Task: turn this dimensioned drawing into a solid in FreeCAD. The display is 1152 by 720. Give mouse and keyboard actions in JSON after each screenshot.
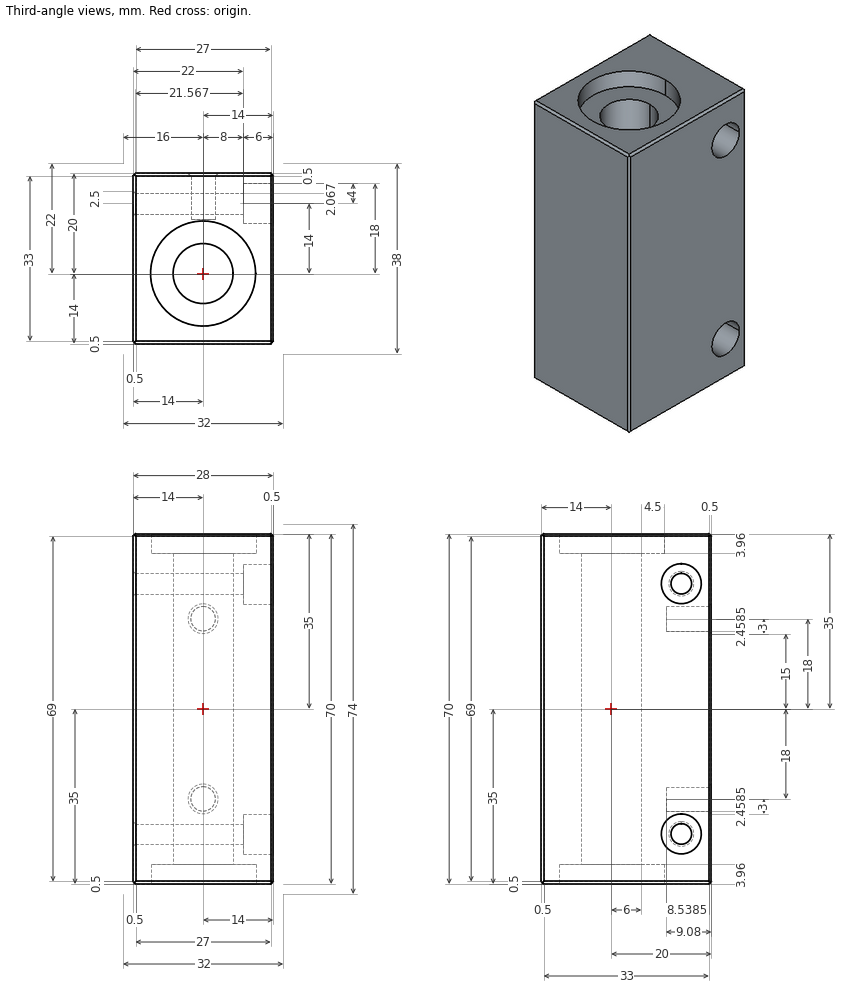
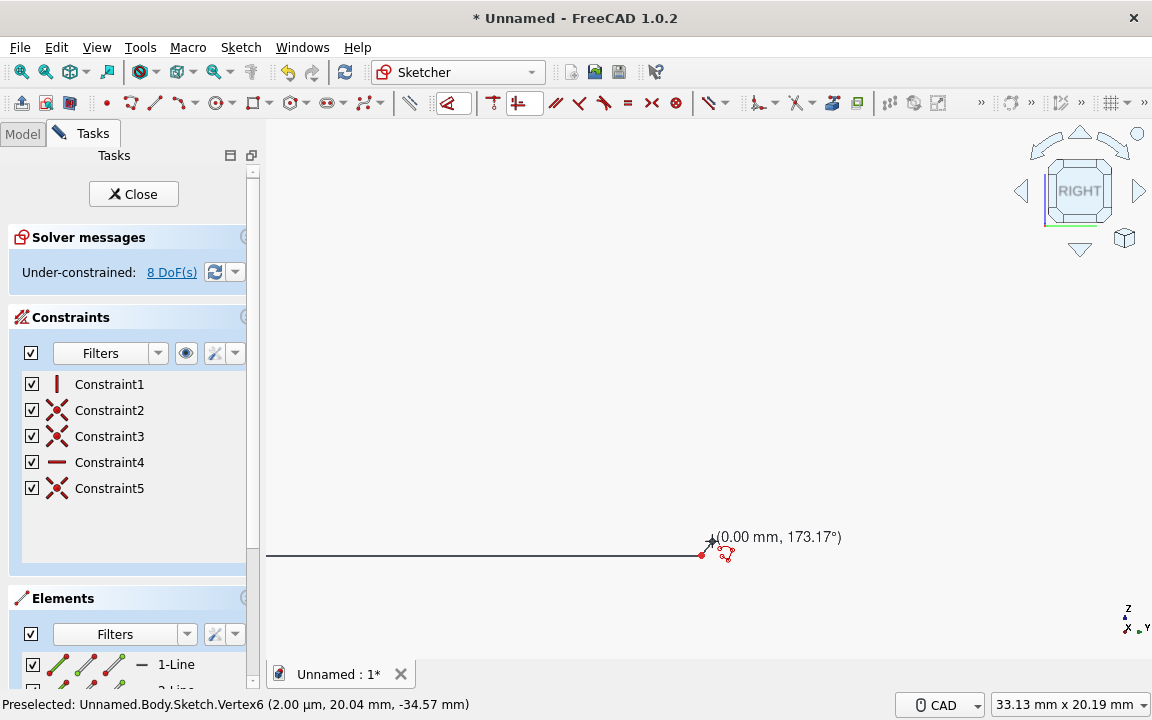
{"action": "scroll", "coordinate": [716, 542], "scroll_direction": "down", "scroll_amount": 9}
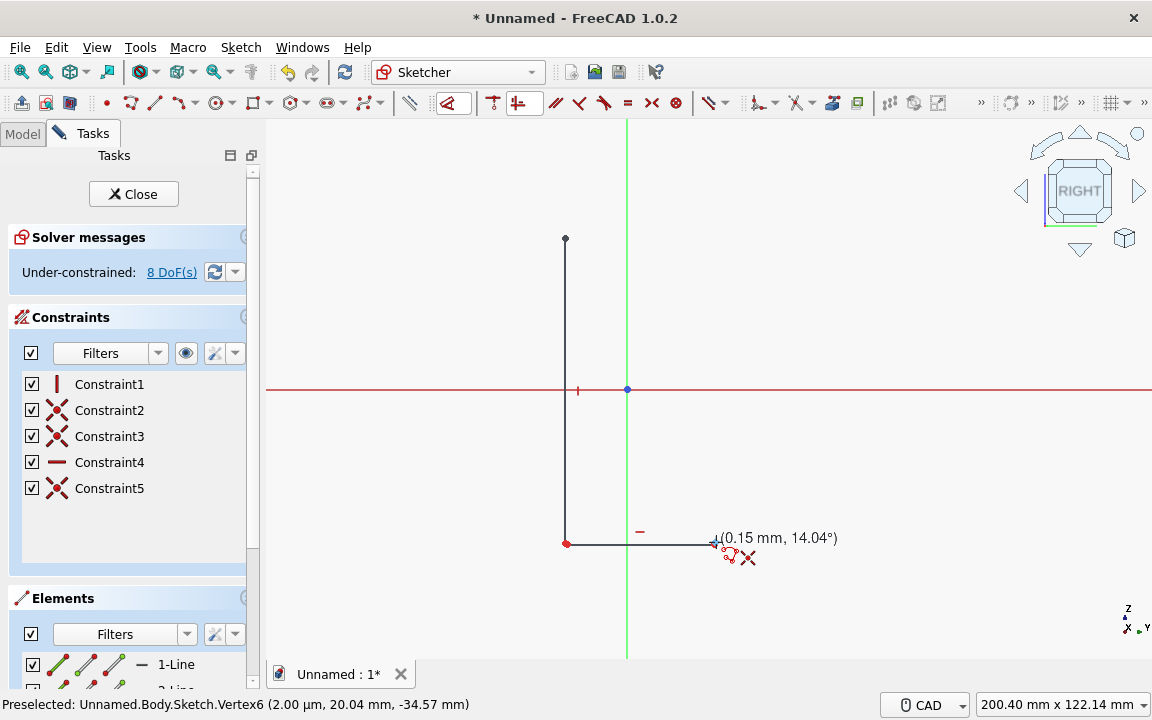
{"action": "left_click", "coordinate": [716, 237]}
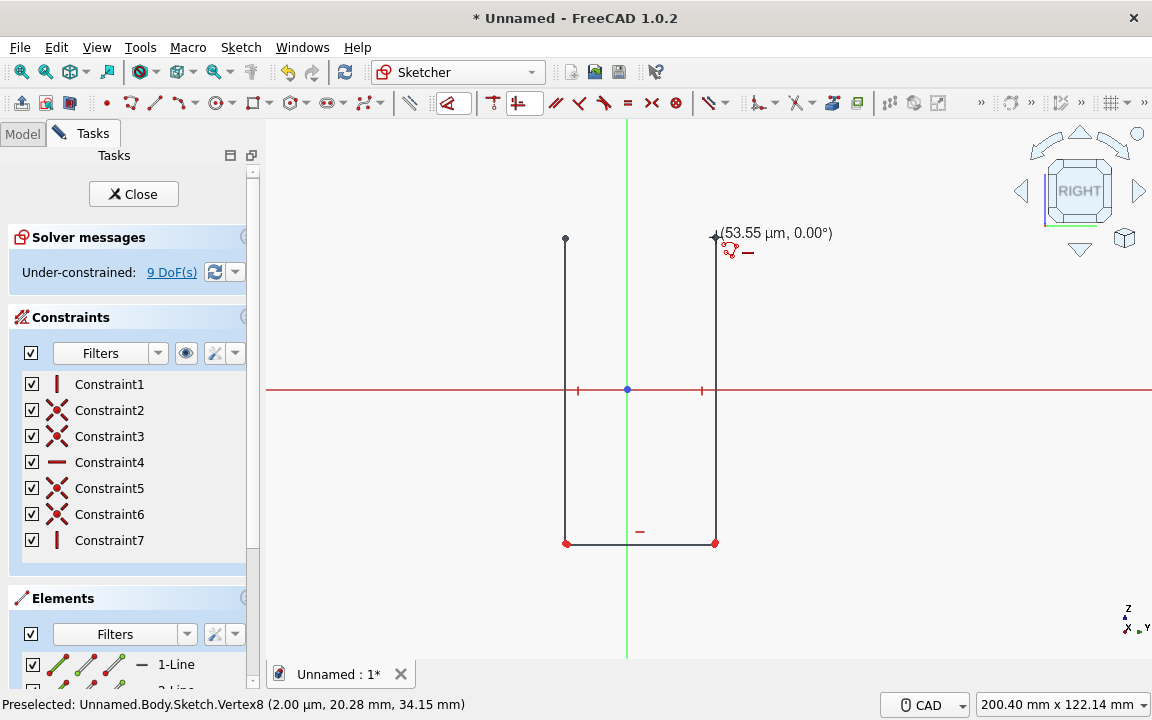
{"action": "scroll", "coordinate": [714, 235], "scroll_direction": "up", "scroll_amount": 9}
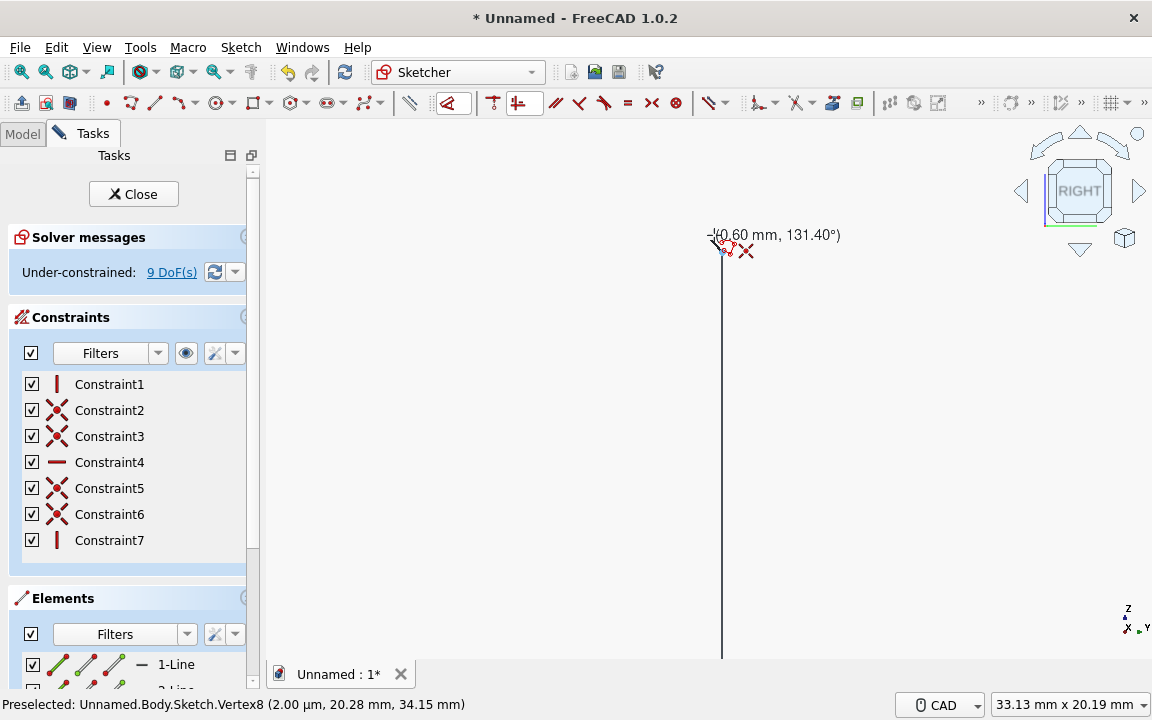
{"action": "left_click", "coordinate": [709, 235]}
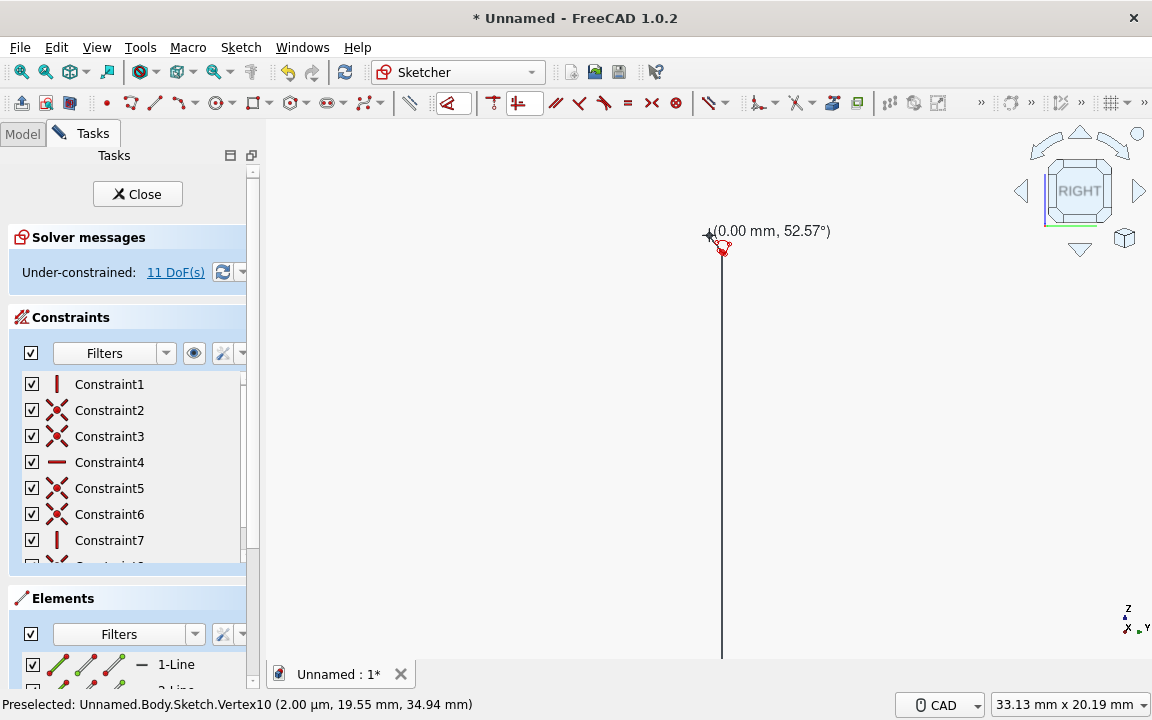
{"action": "scroll", "coordinate": [714, 234], "scroll_direction": "down", "scroll_amount": 9}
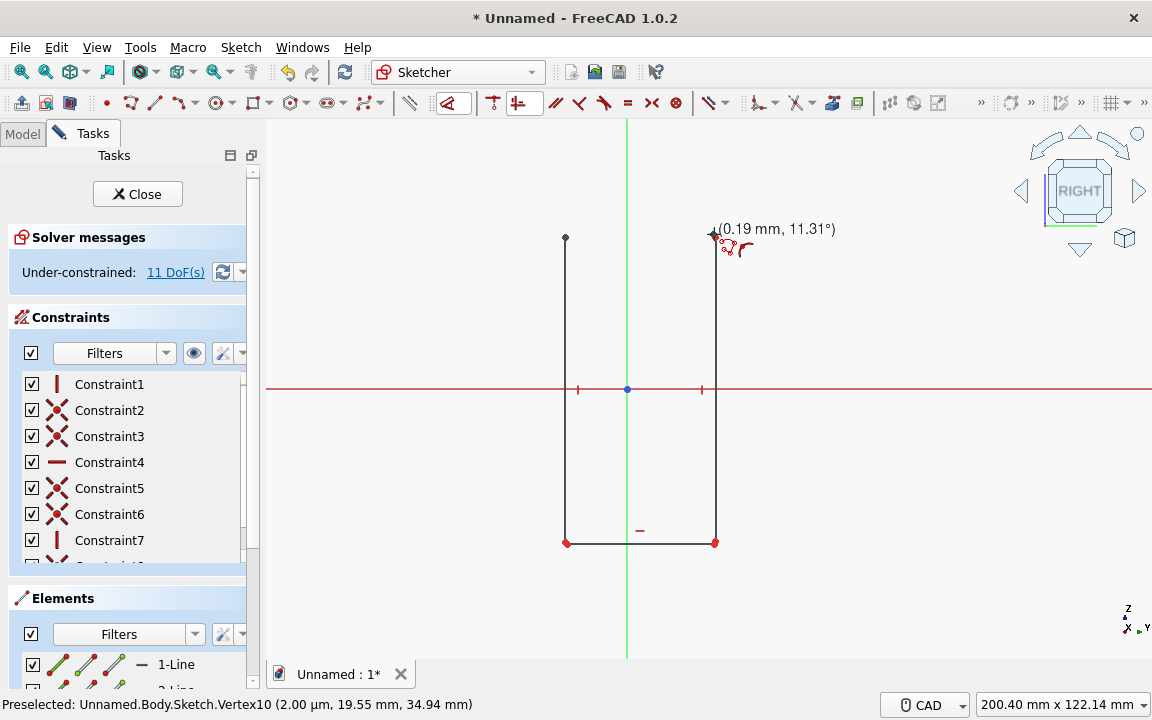
{"action": "scroll", "coordinate": [568, 234], "scroll_direction": "up", "scroll_amount": 9}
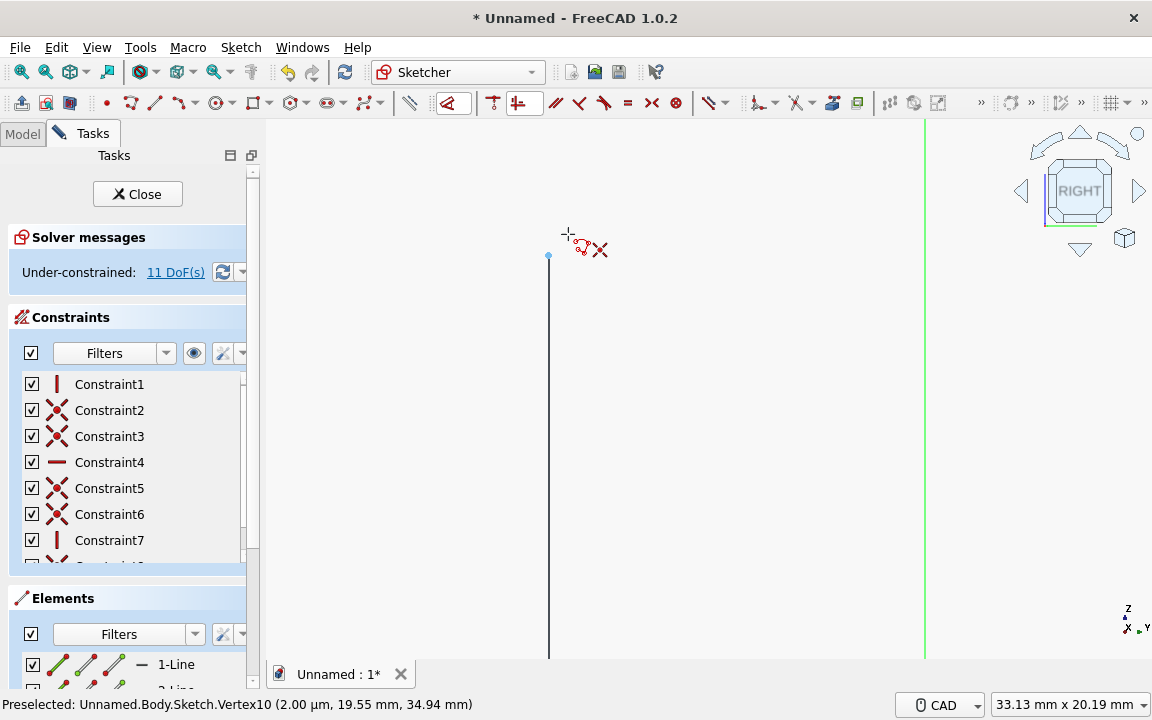
{"action": "left_click", "coordinate": [564, 235]}
{"action": "left_click", "coordinate": [549, 255]}
{"action": "key", "text": "Escape"}
{"action": "key", "text": "Escape"}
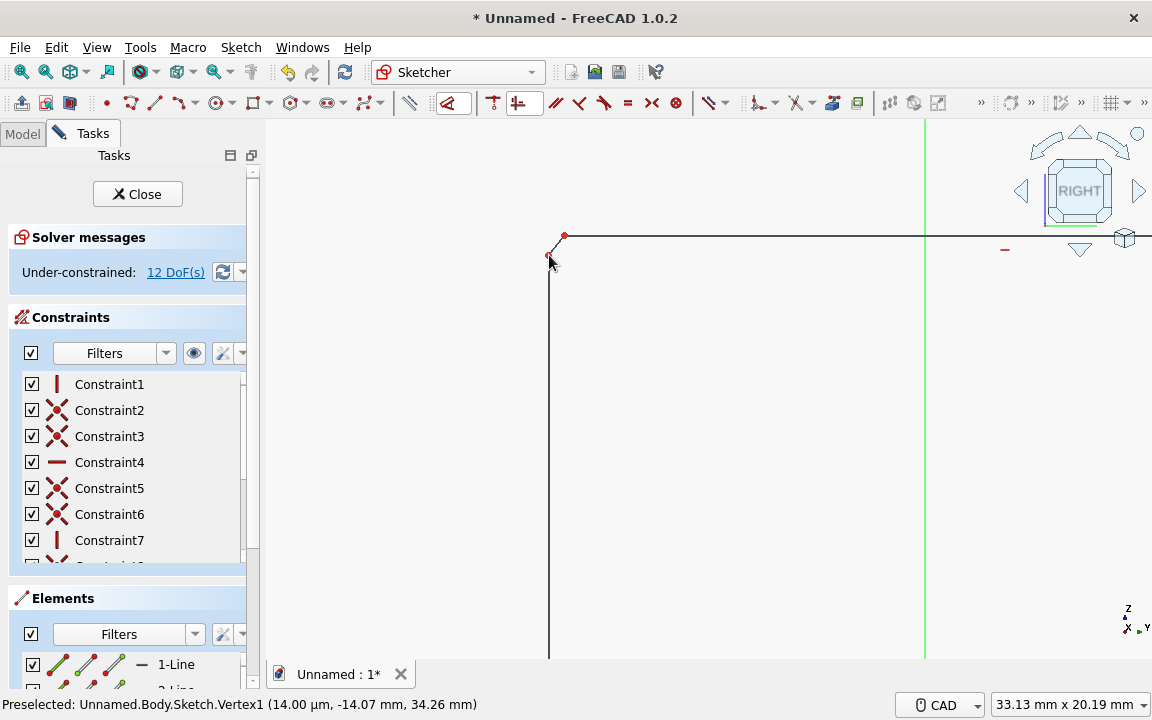
{"action": "left_click", "coordinate": [448, 104]}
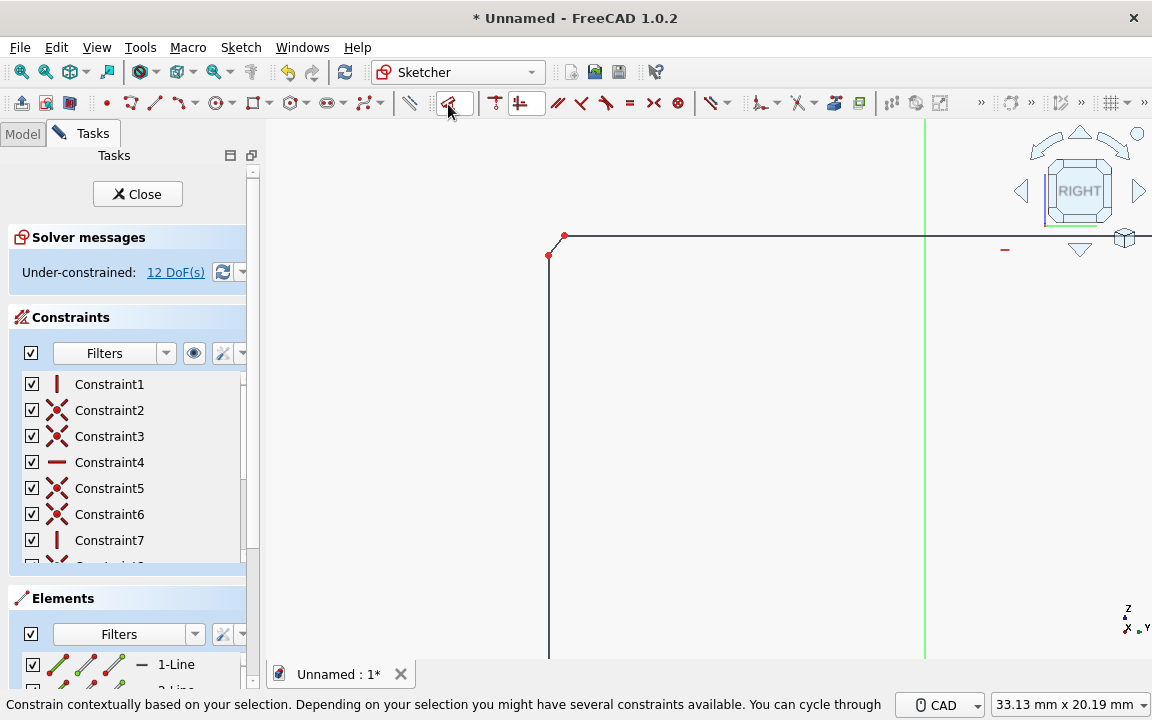
{"action": "scroll", "coordinate": [568, 234], "scroll_direction": "down", "scroll_amount": 9}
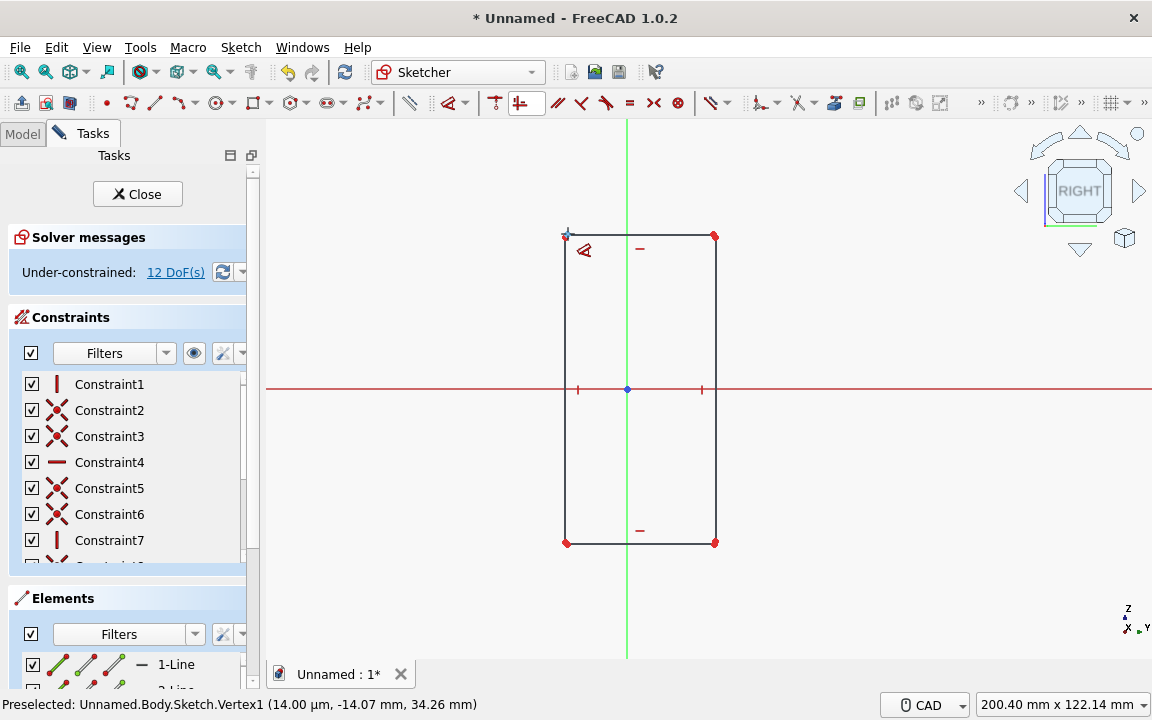
{"action": "left_click", "coordinate": [565, 299]}
{"action": "left_click", "coordinate": [531, 320]}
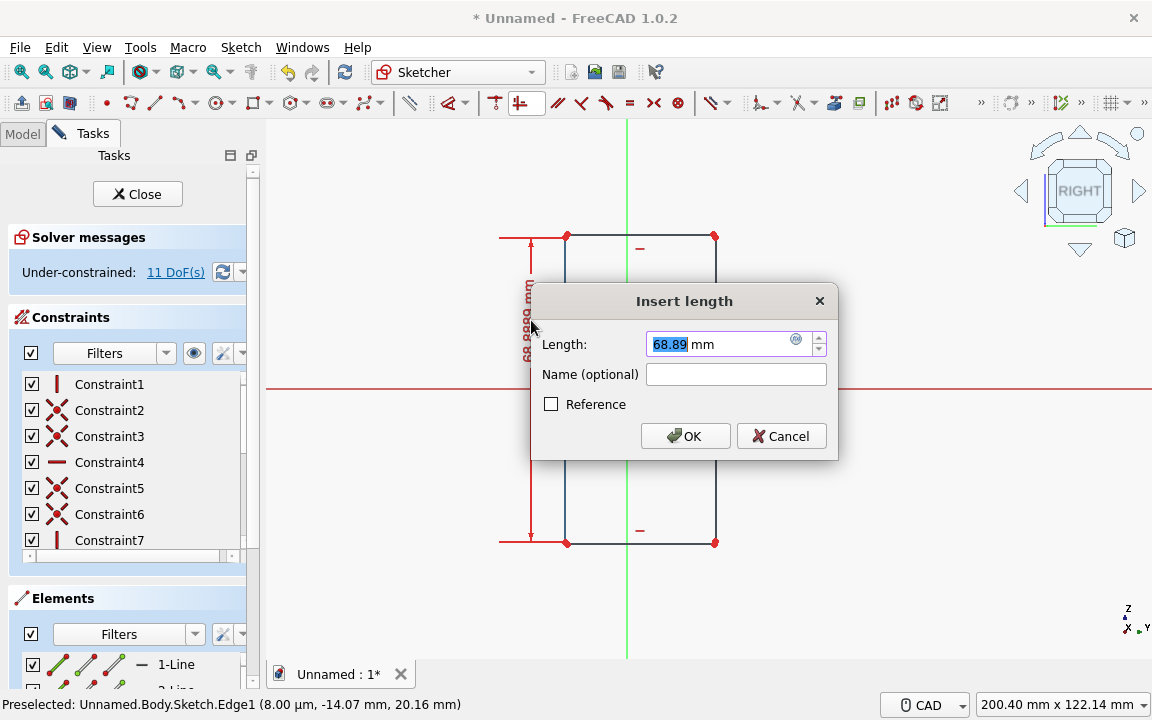
{"action": "type", "text": "69"}
{"action": "key", "text": "Return"}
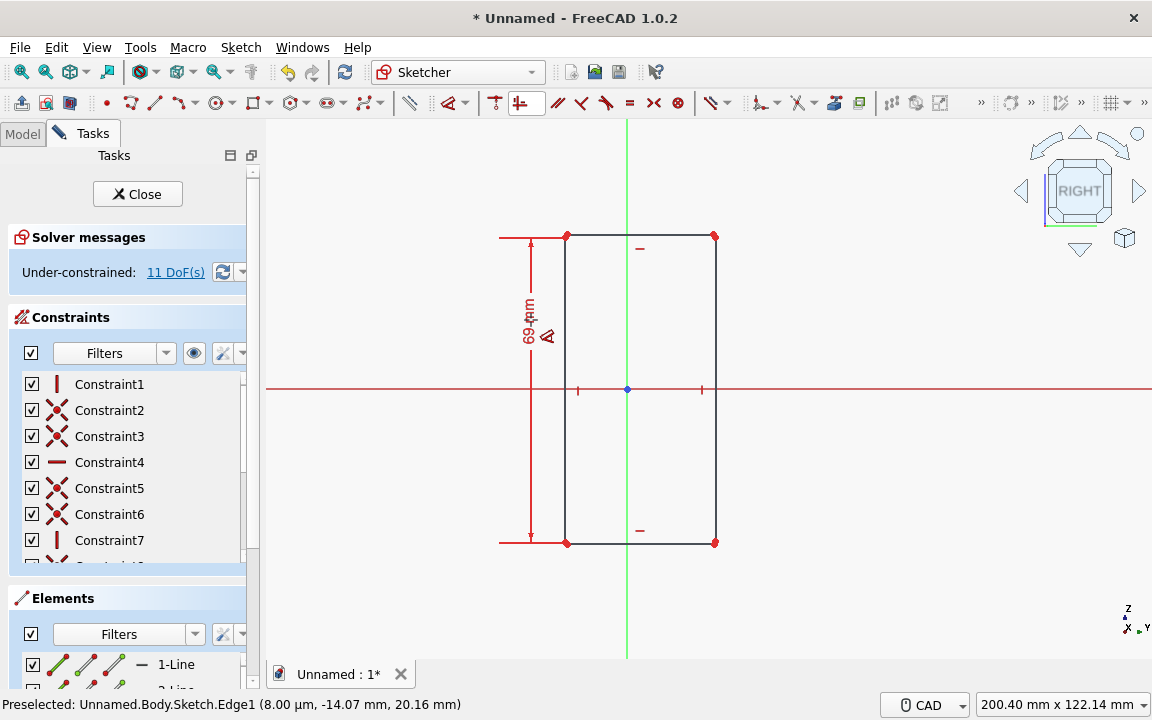
{"action": "left_click", "coordinate": [612, 544]}
{"action": "left_click", "coordinate": [641, 578]}